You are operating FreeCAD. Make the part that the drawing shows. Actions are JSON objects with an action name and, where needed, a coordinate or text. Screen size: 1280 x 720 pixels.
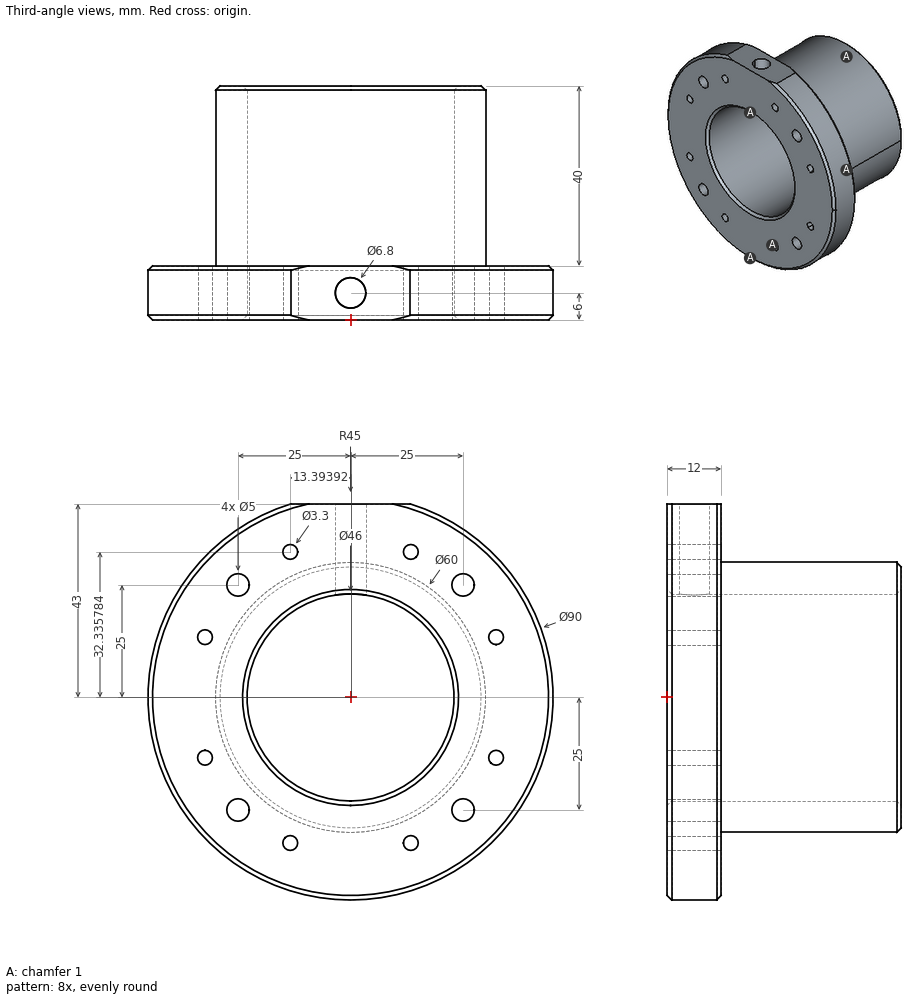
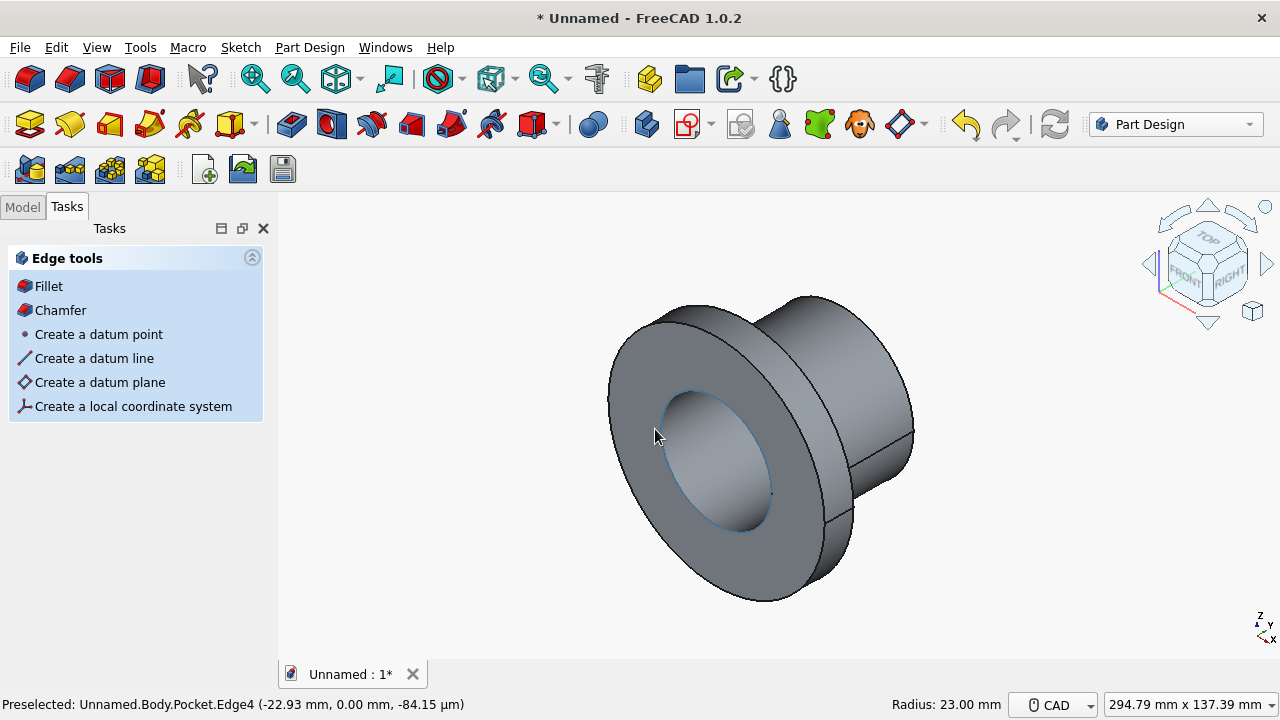
{"action": "left_click", "coordinate": [683, 323], "text": "ctrl"}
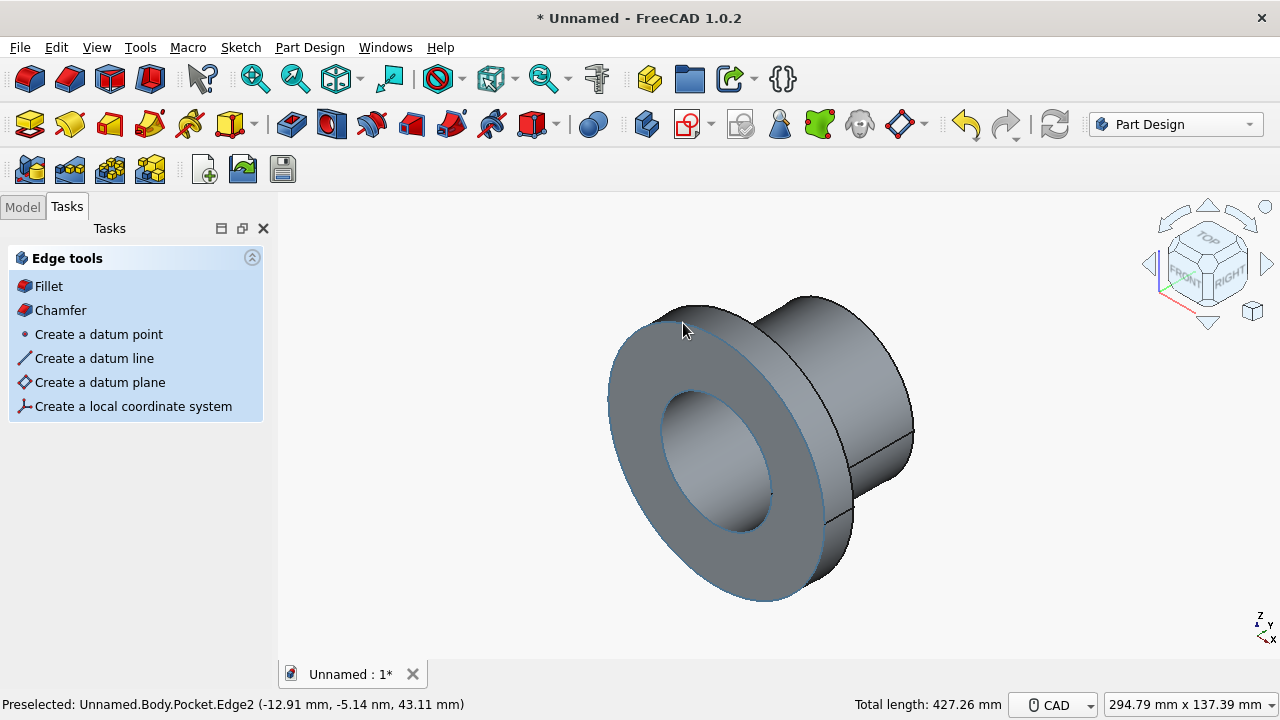
{"action": "left_click", "coordinate": [819, 296], "text": "ctrl"}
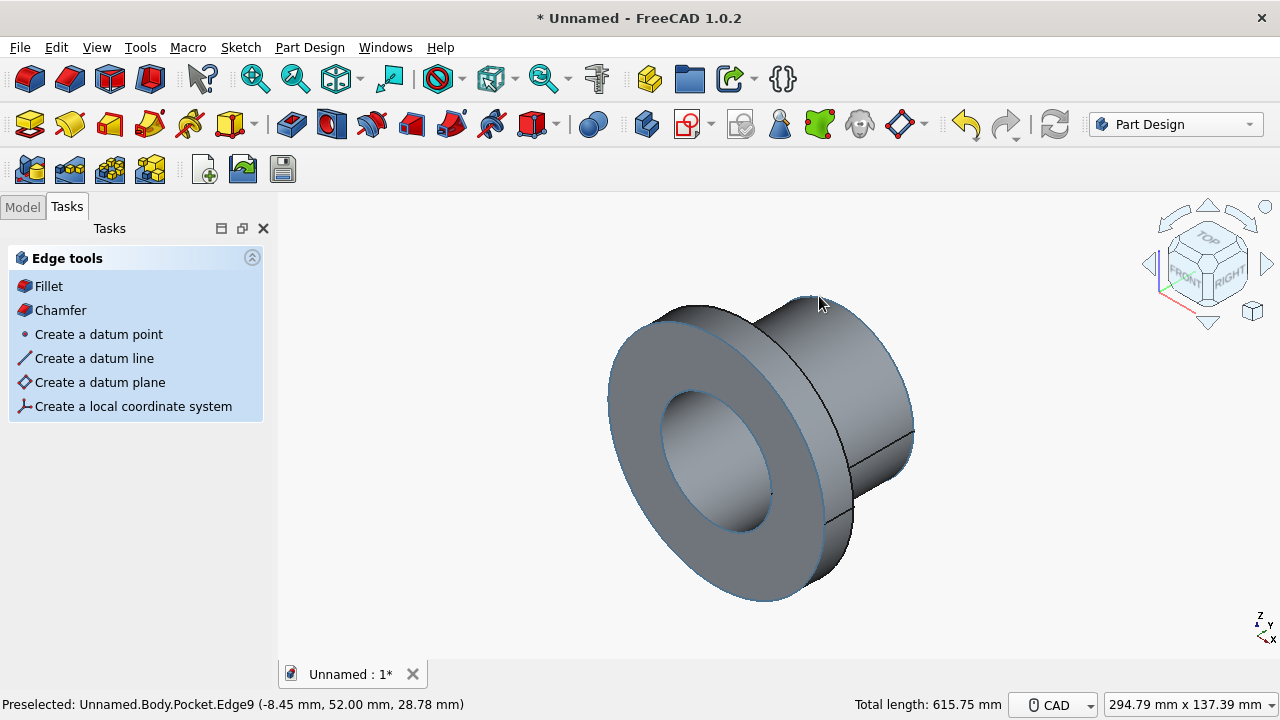
{"action": "key", "text": "2"}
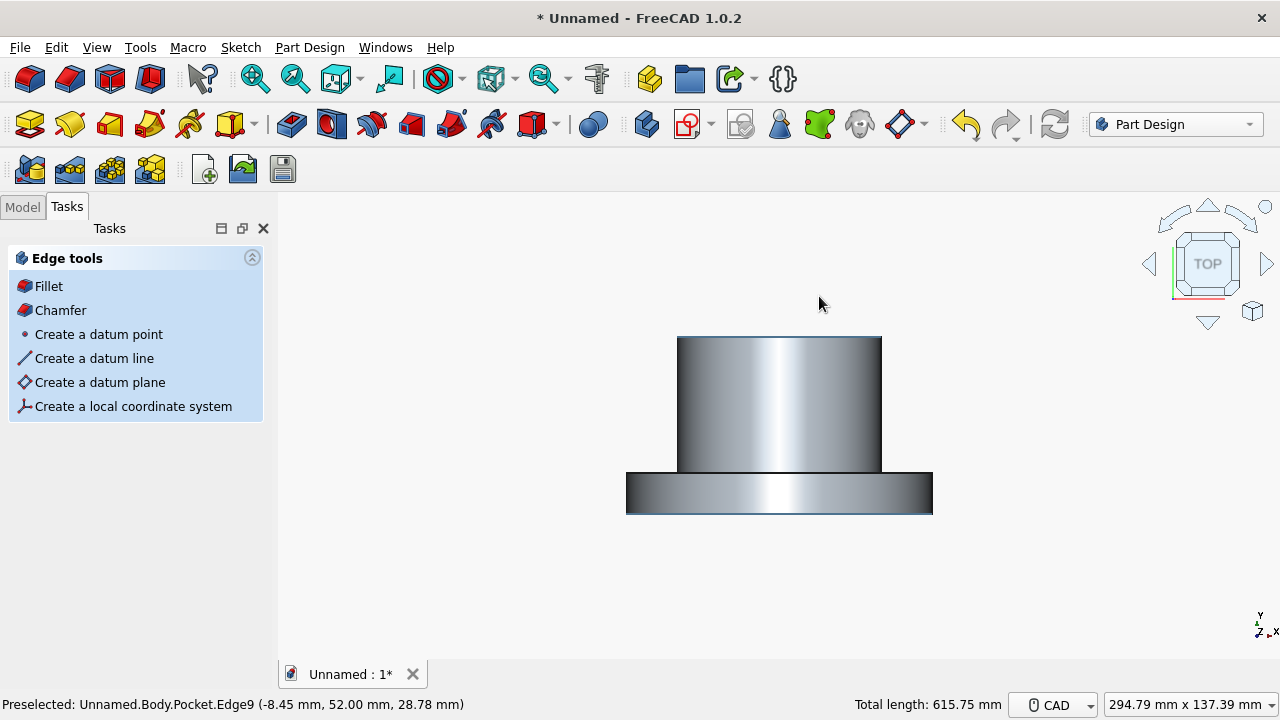
{"action": "key", "text": "v f"}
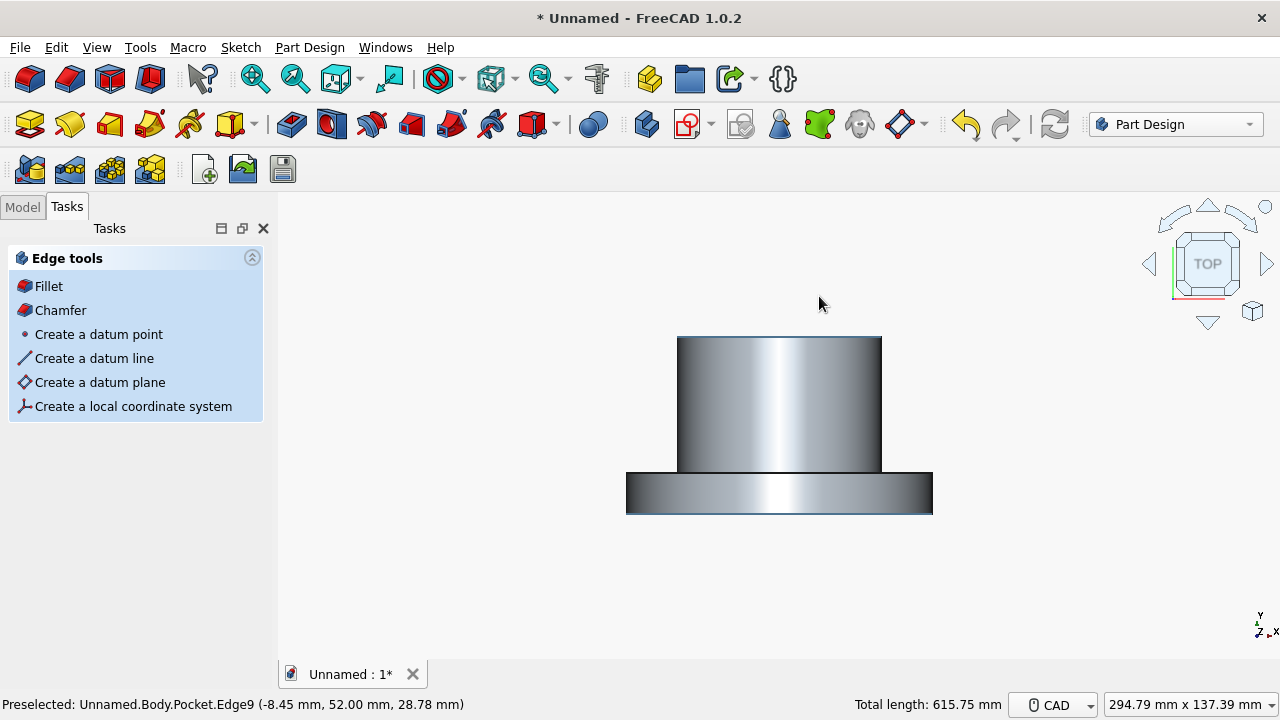
{"action": "left_click", "coordinate": [655, 472], "text": "ctrl"}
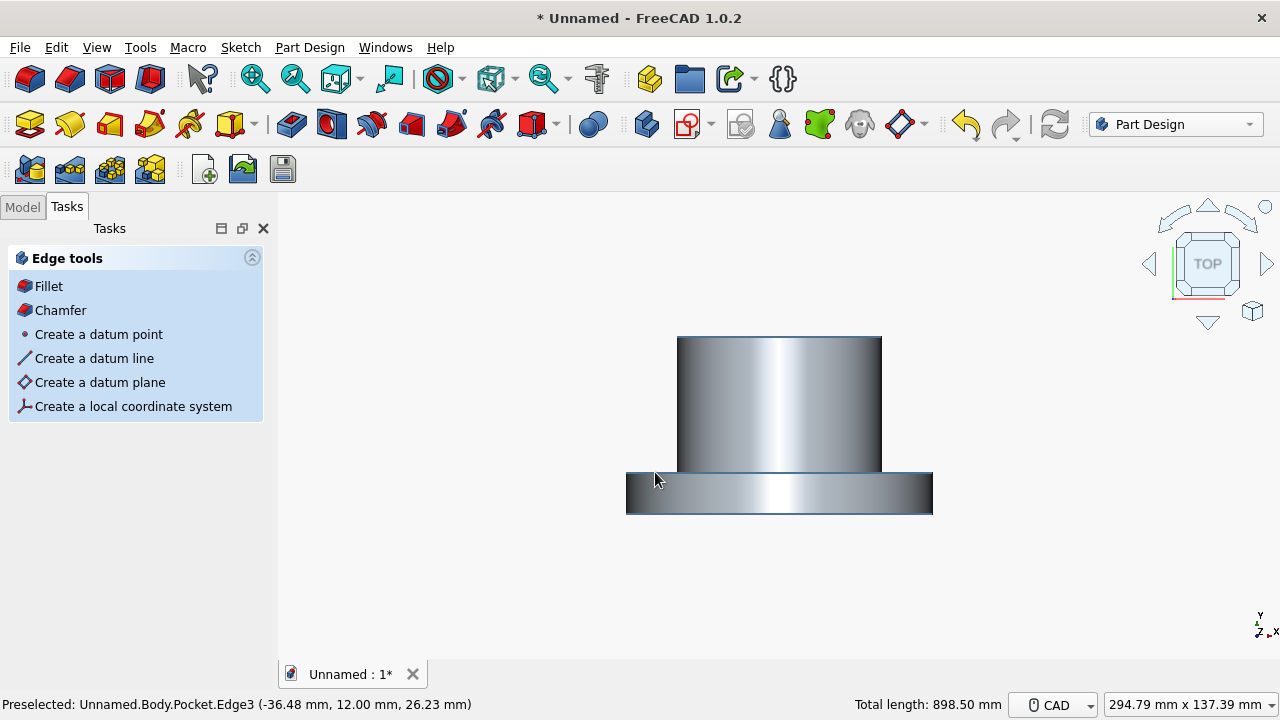
{"action": "key", "text": "0"}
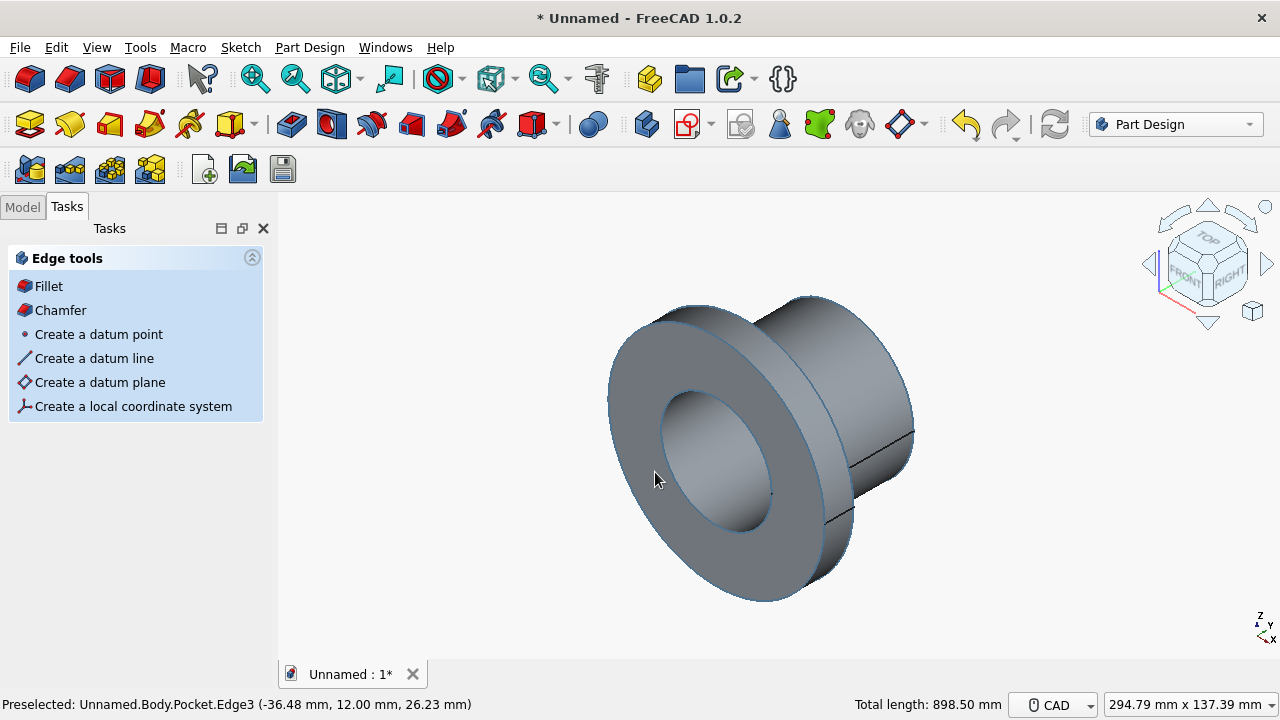
{"action": "key", "text": "1"}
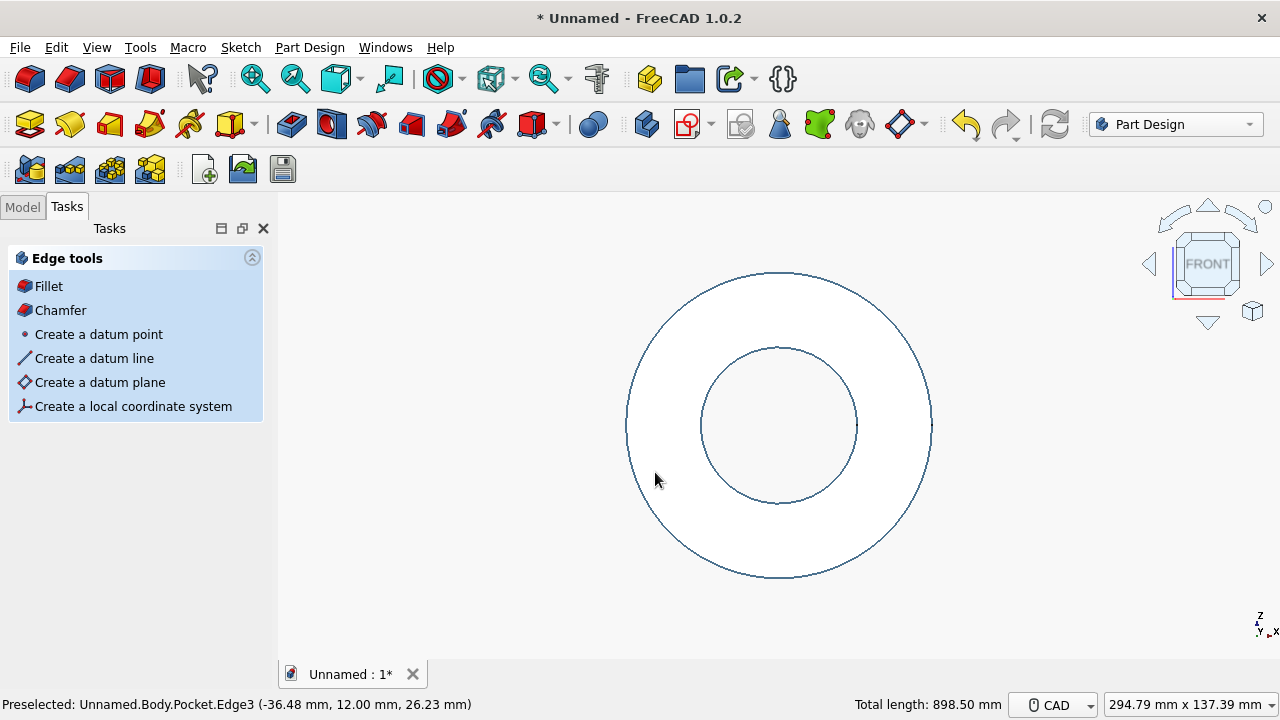
{"action": "key", "text": "3"}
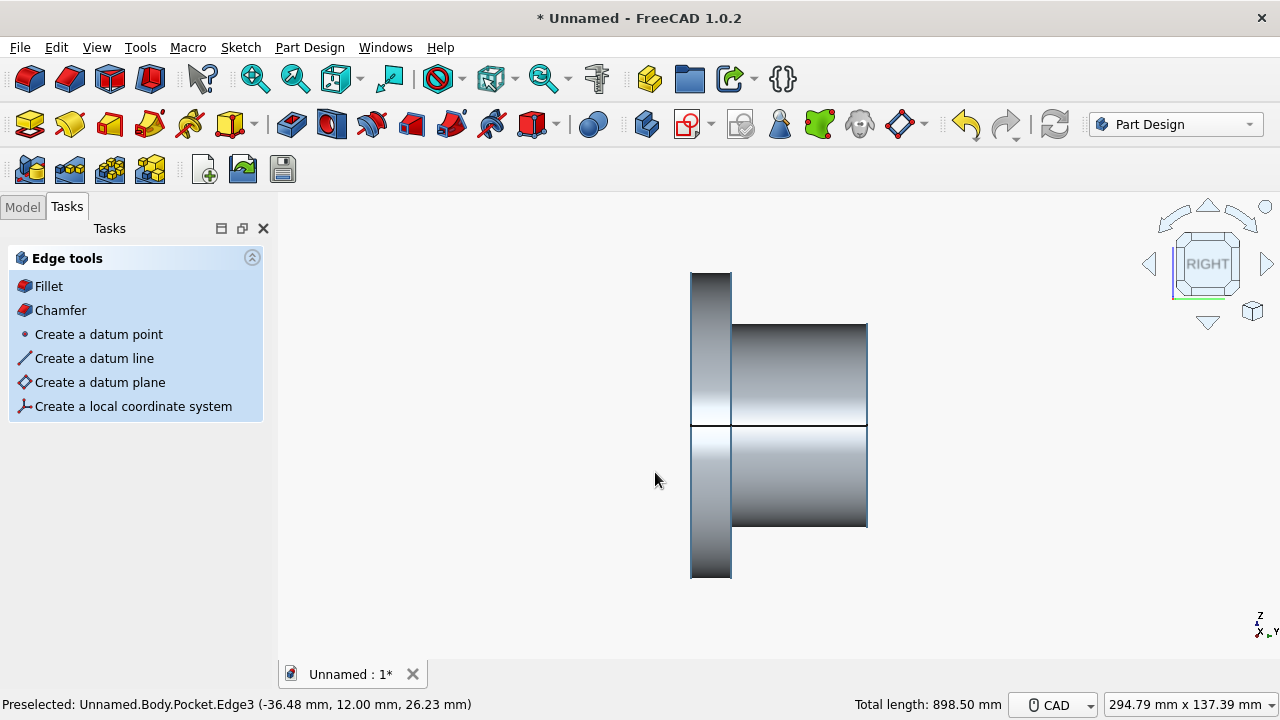
{"action": "key", "text": "5"}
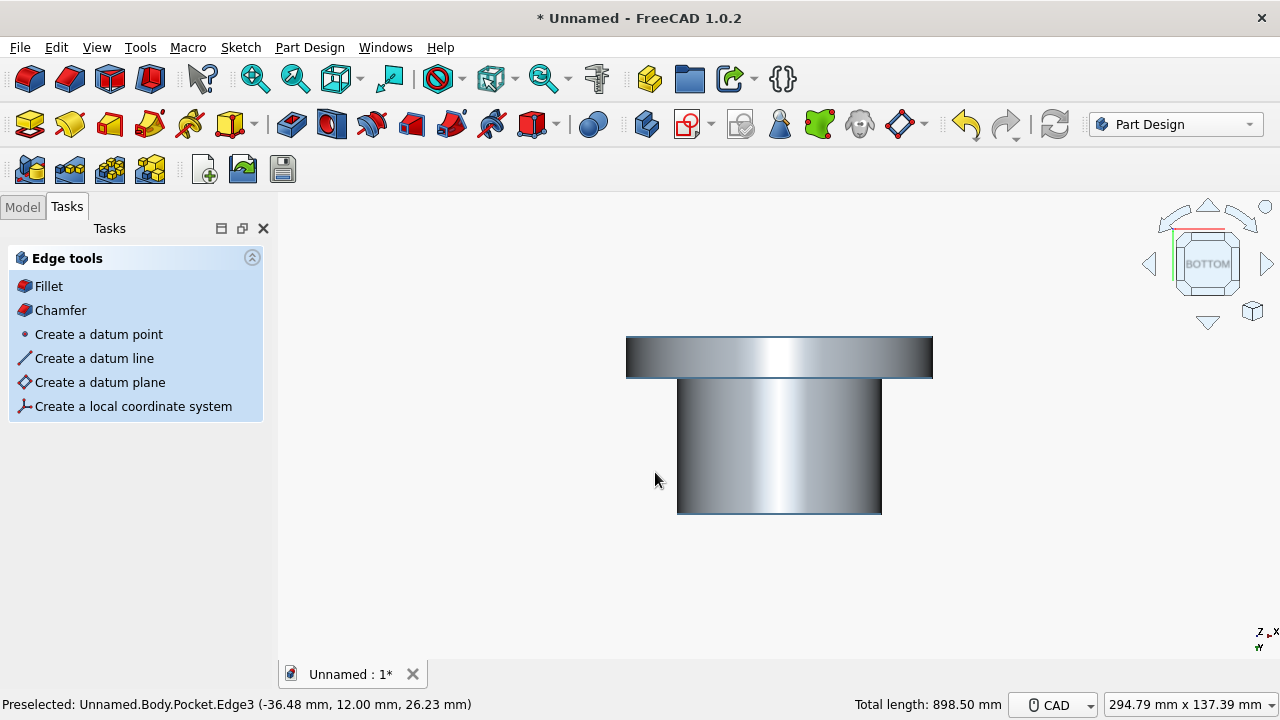
{"action": "left_click", "coordinate": [256, 80]}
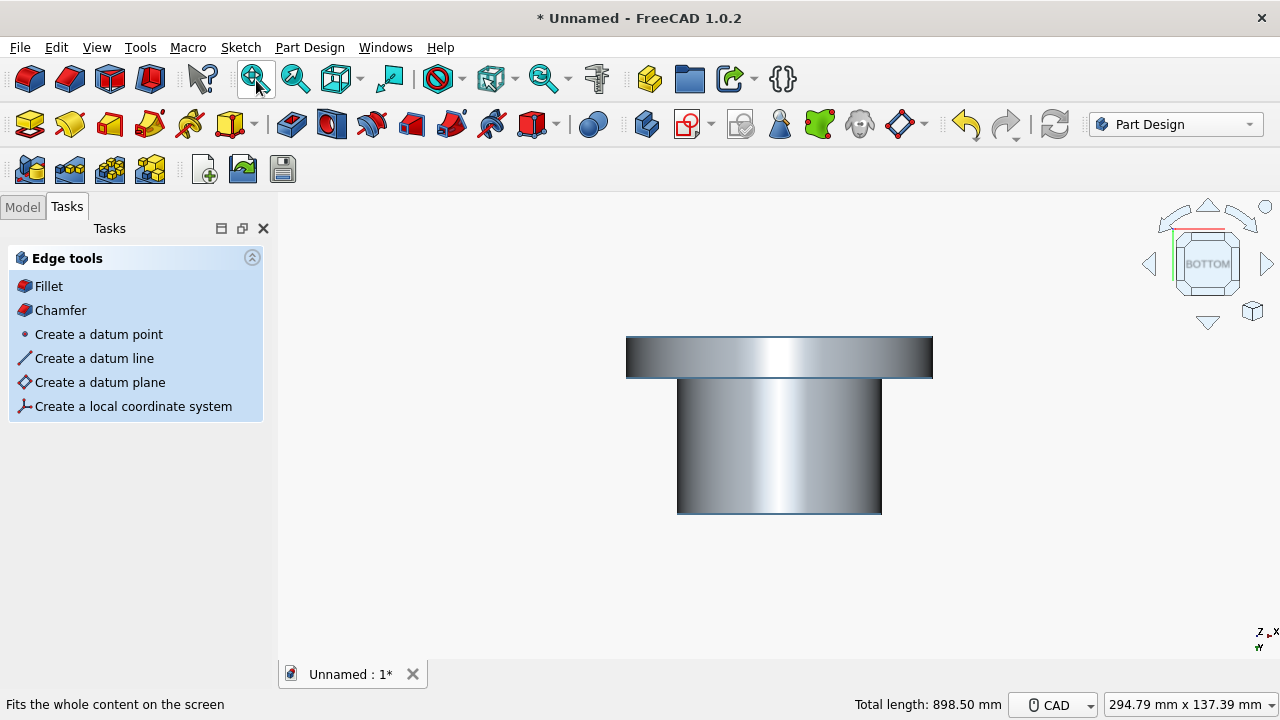
{"action": "key", "text": "4"}